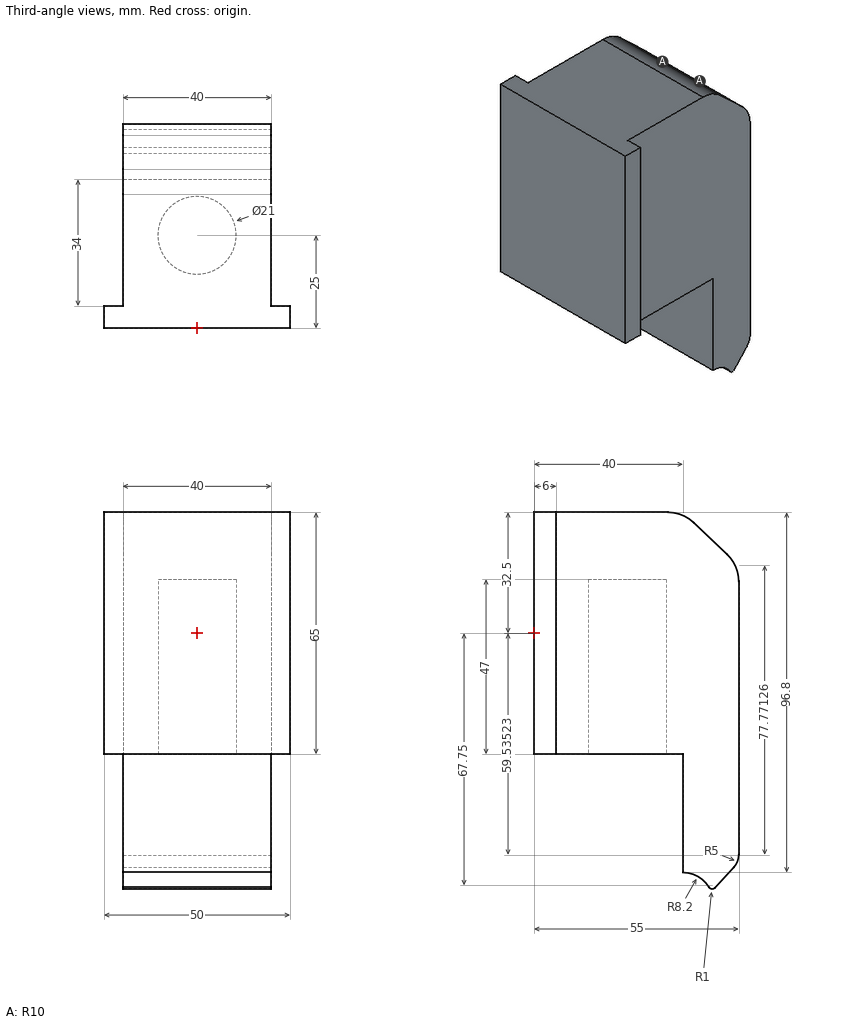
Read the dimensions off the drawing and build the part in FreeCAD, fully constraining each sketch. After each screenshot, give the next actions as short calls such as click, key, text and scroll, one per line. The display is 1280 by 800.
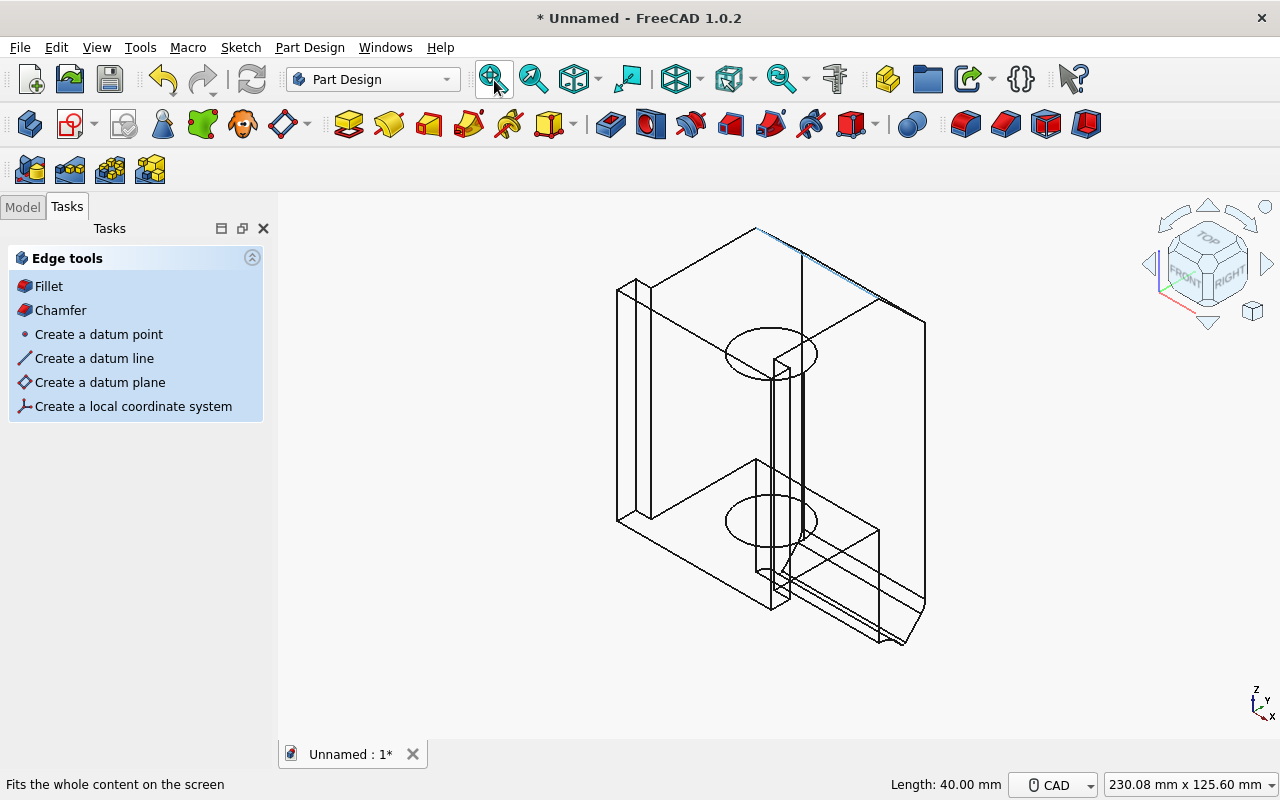
key(2)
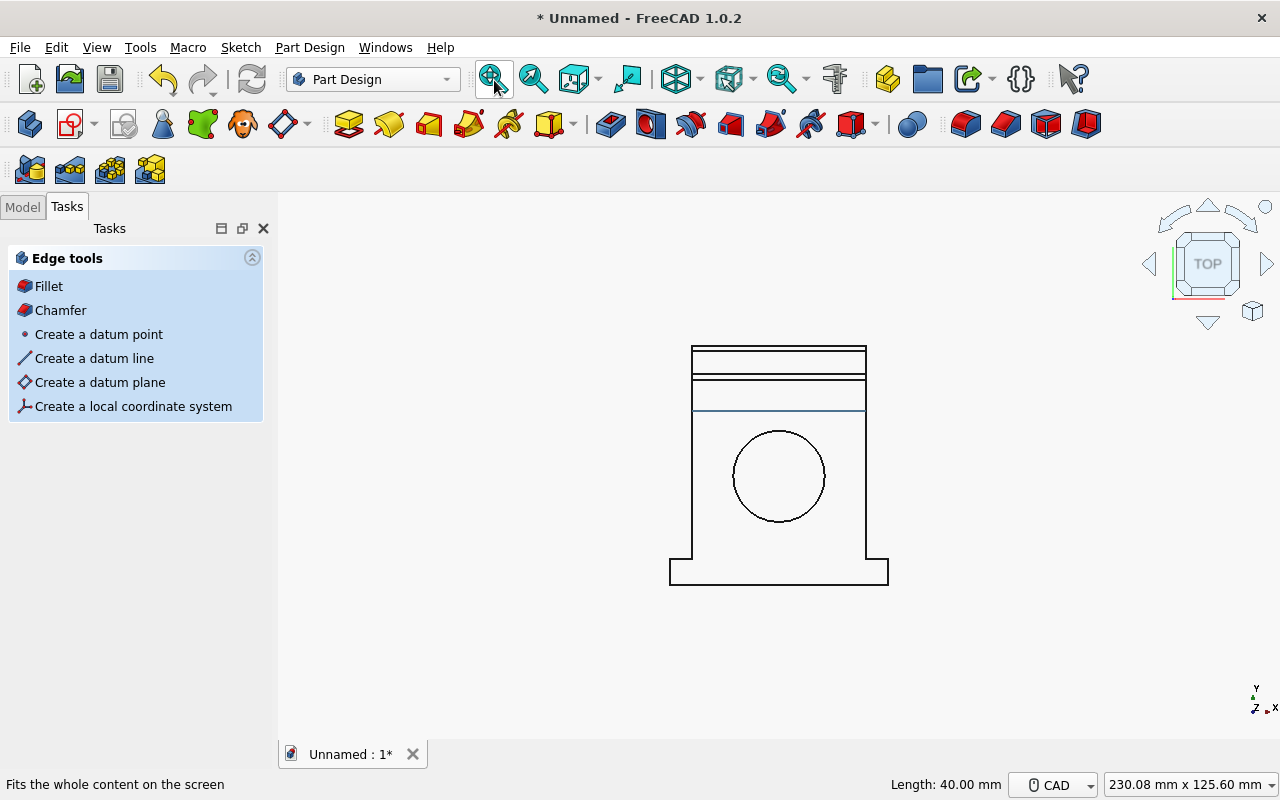
key(v)
key(f)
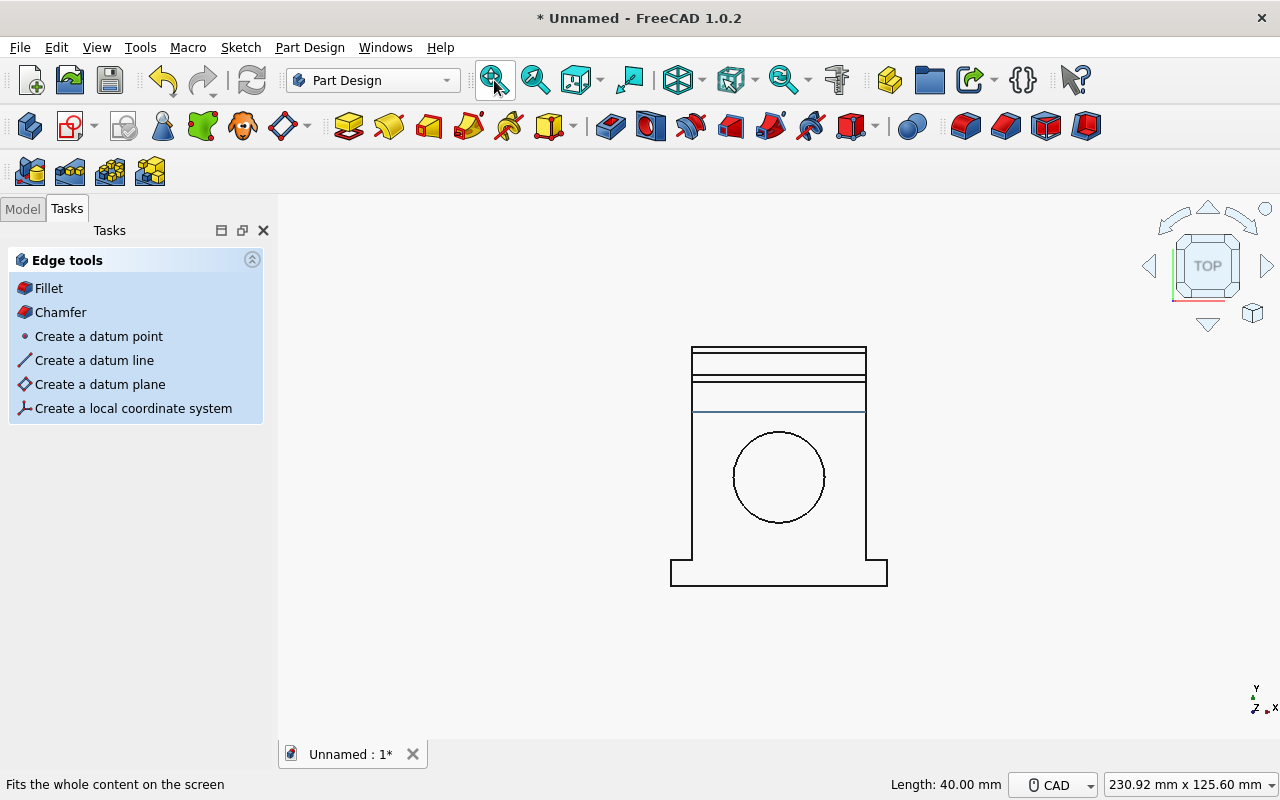
click(779, 346, ctrl)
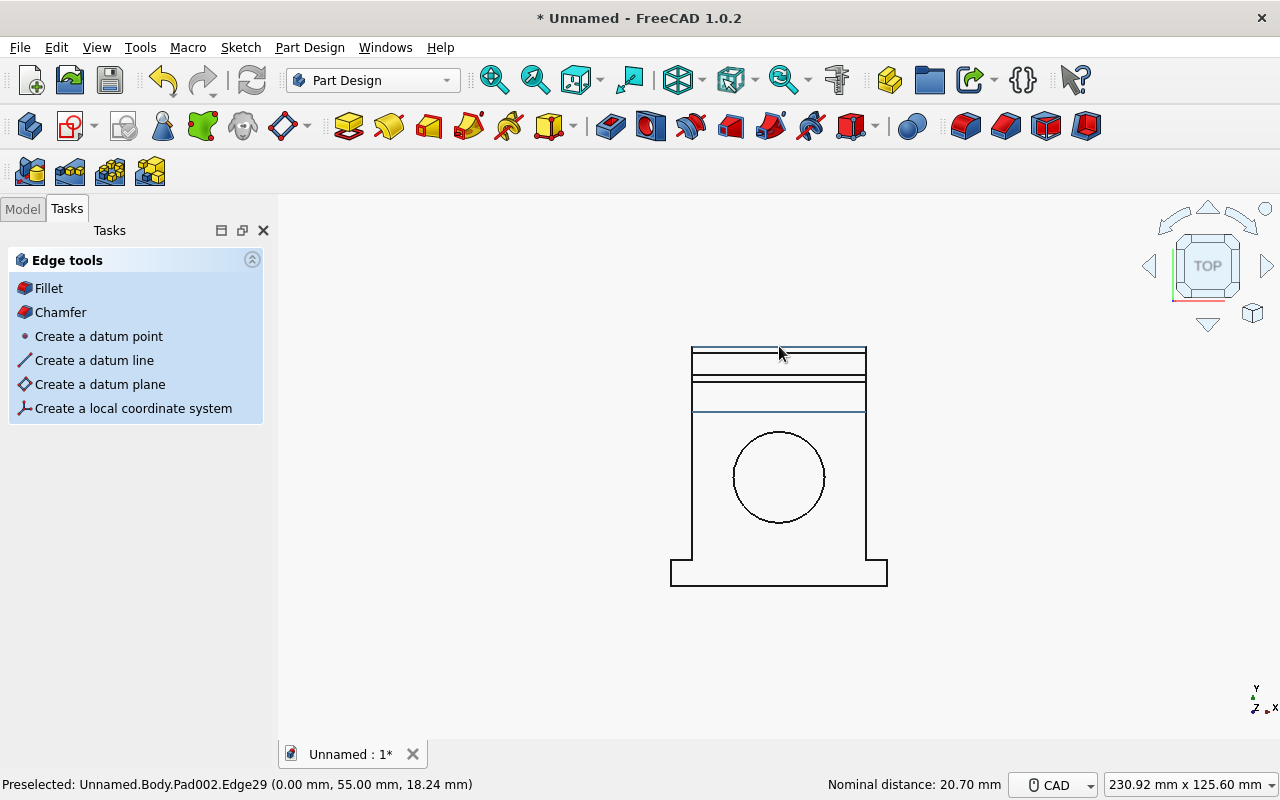
key(v)
key(1)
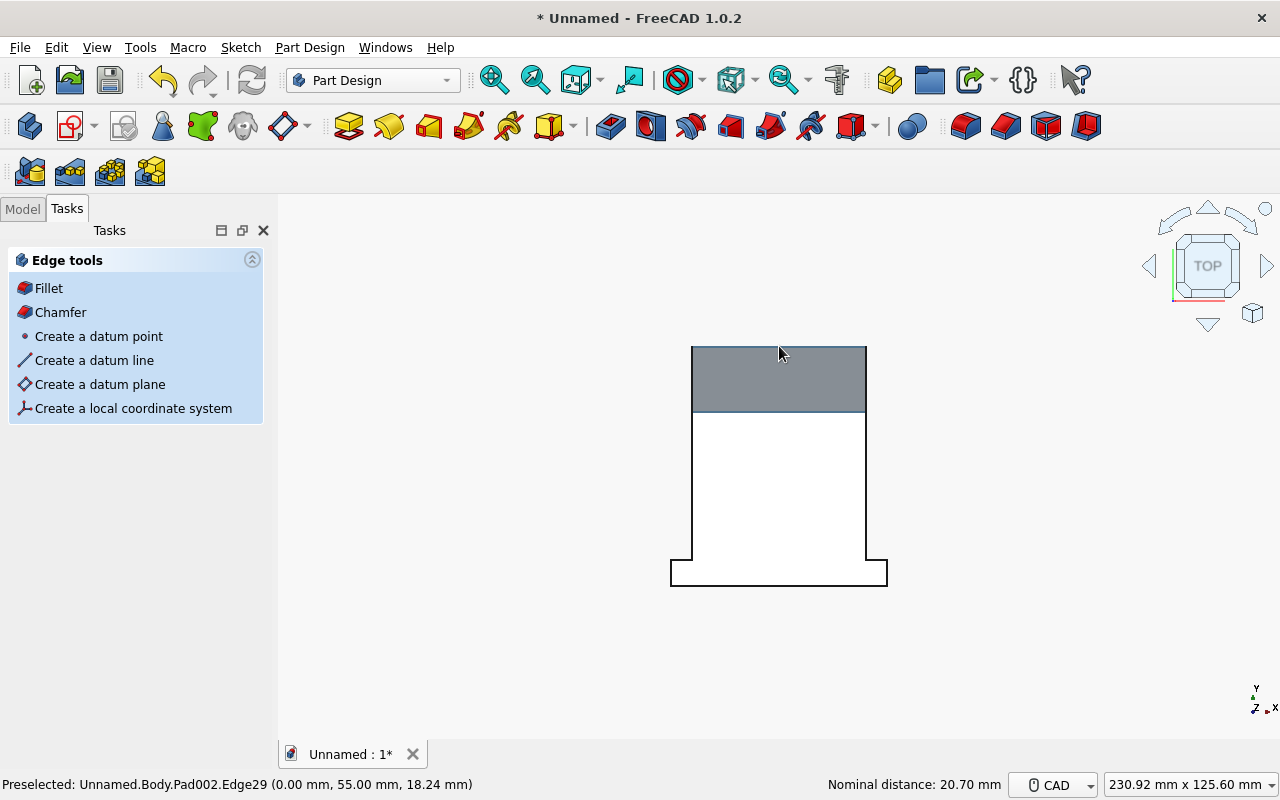
click(966, 126)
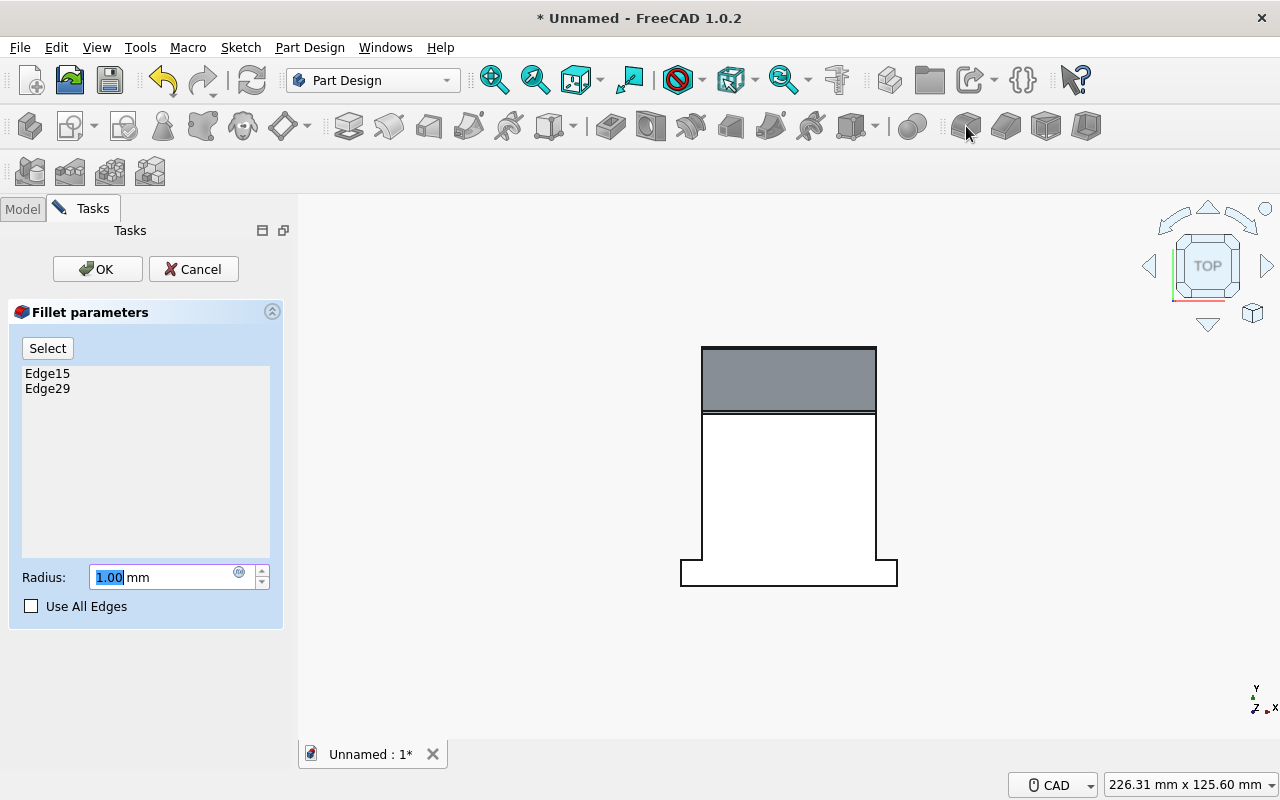
text(10)
key(Tab)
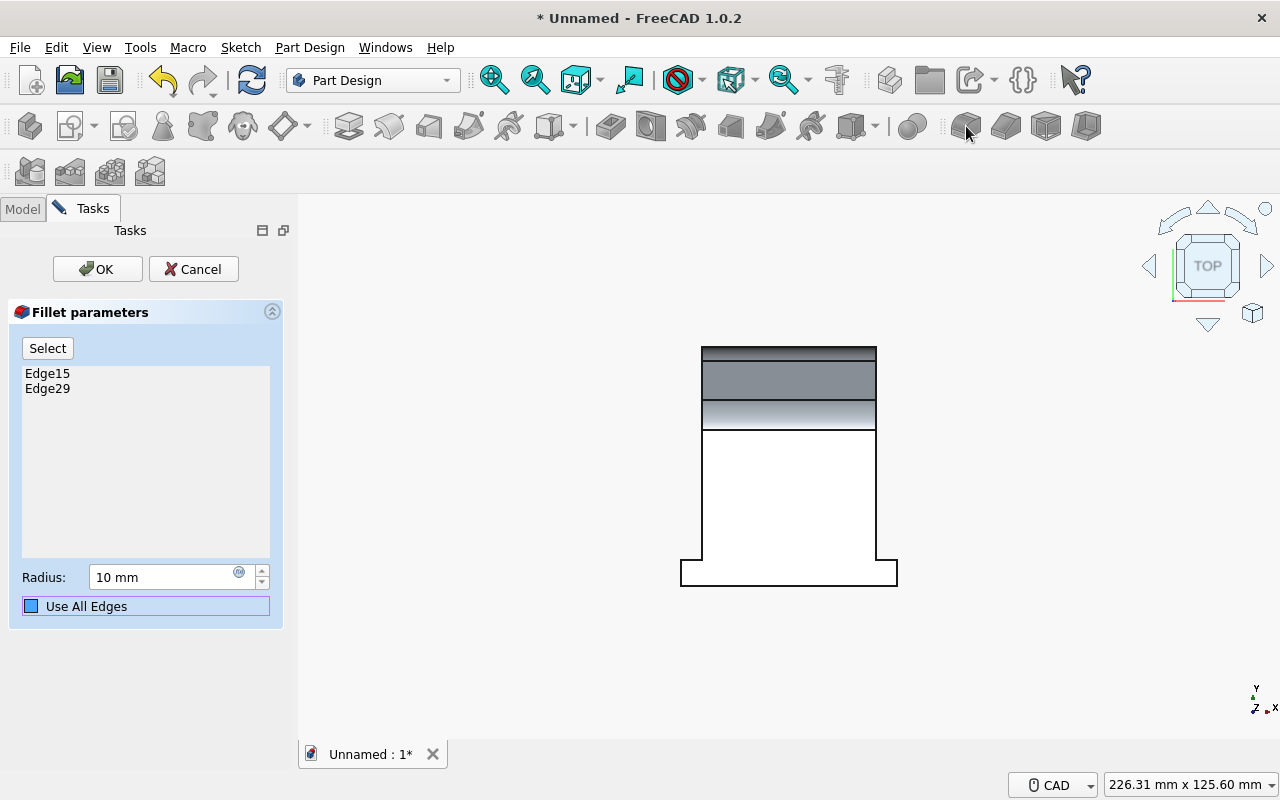
click(98, 269)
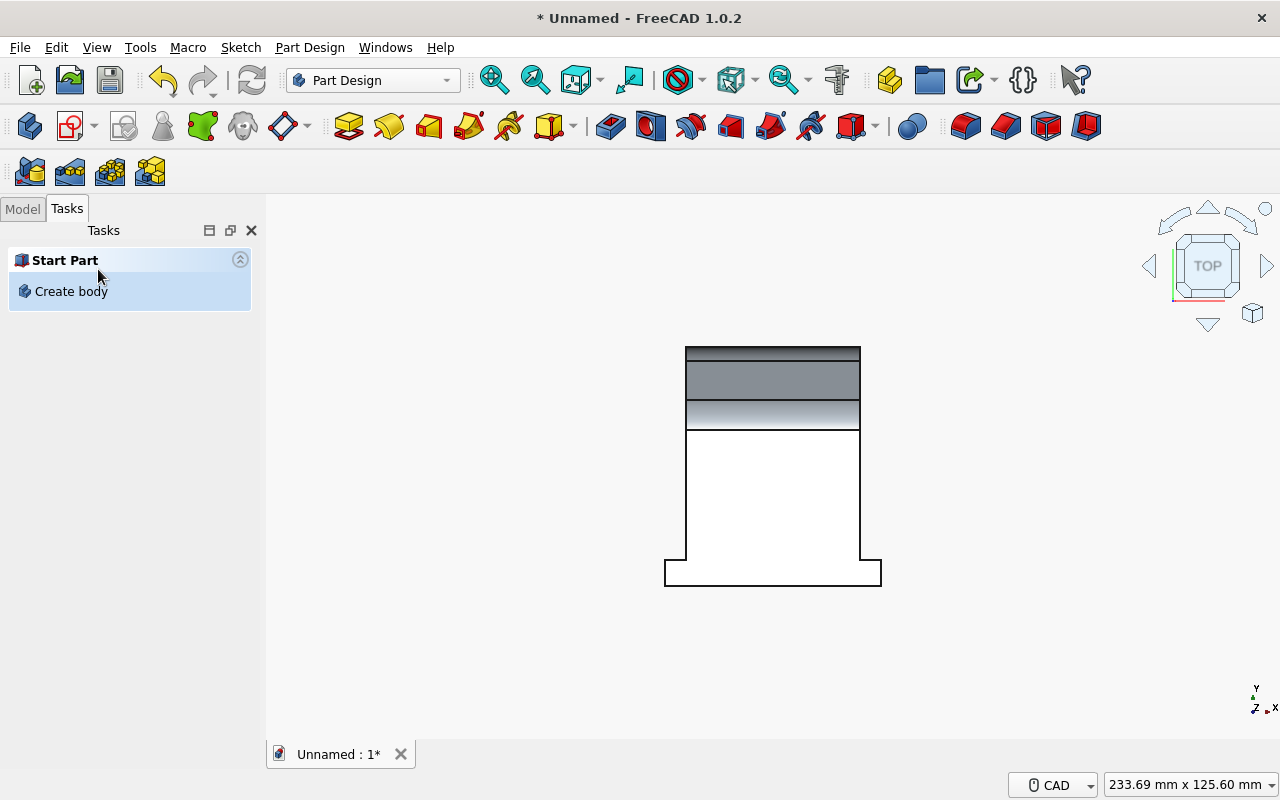
key(0)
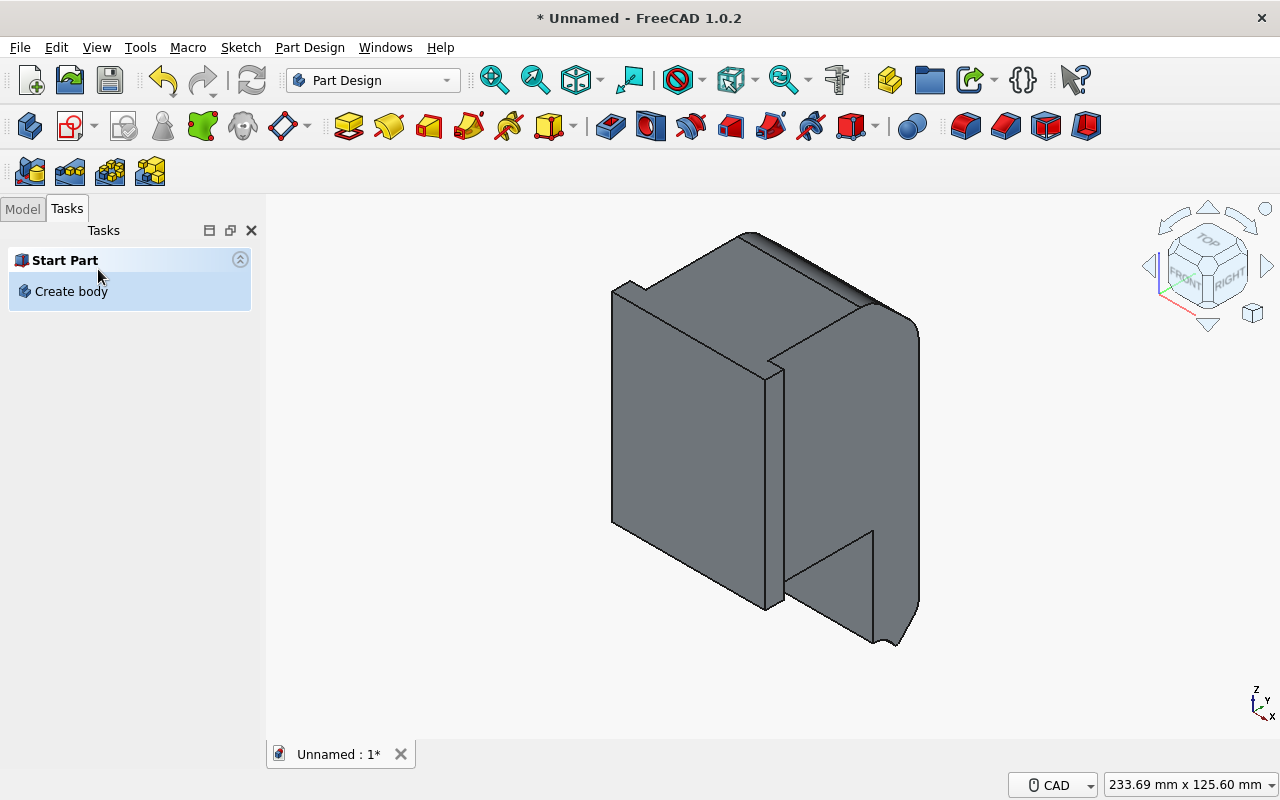
click(496, 80)